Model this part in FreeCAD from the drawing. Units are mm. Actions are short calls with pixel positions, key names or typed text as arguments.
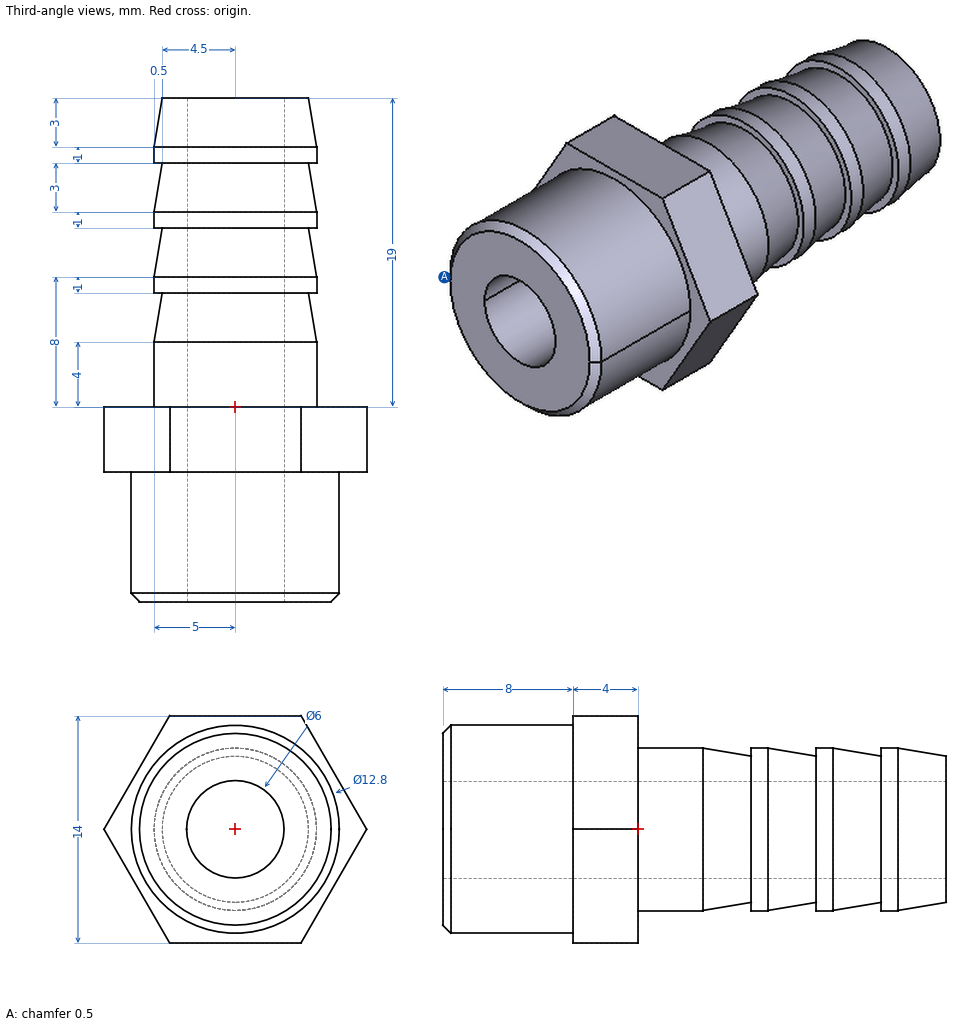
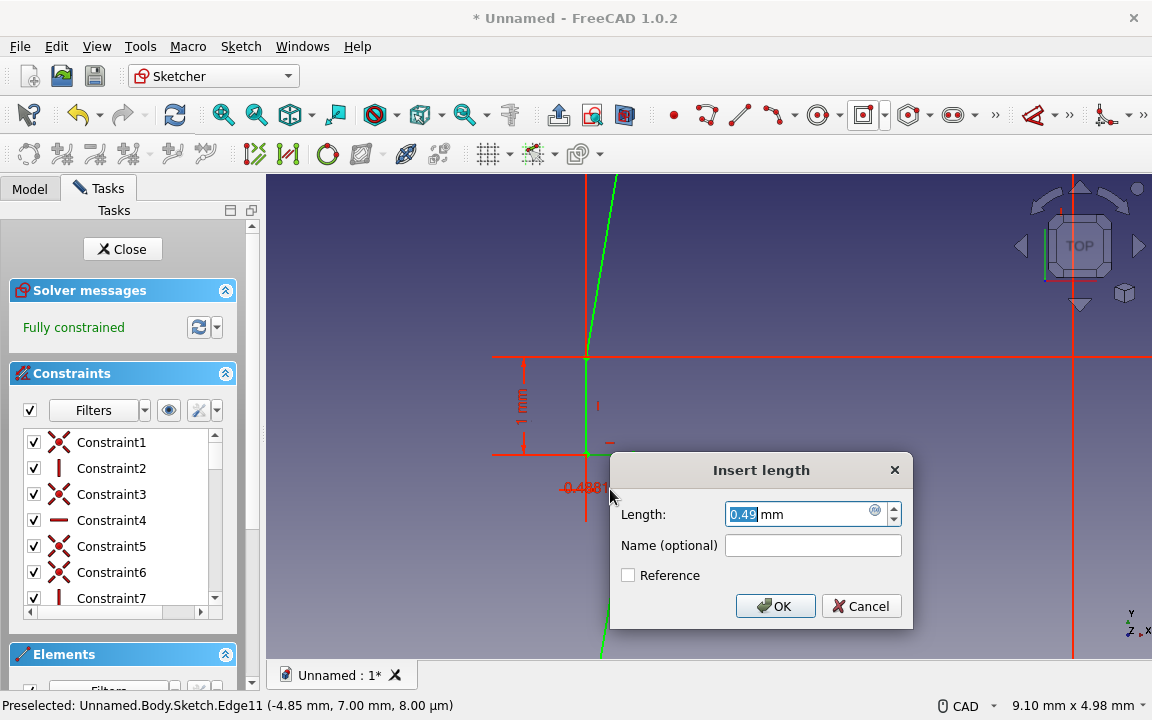
text(0.5)
key(Return)
key(Escape)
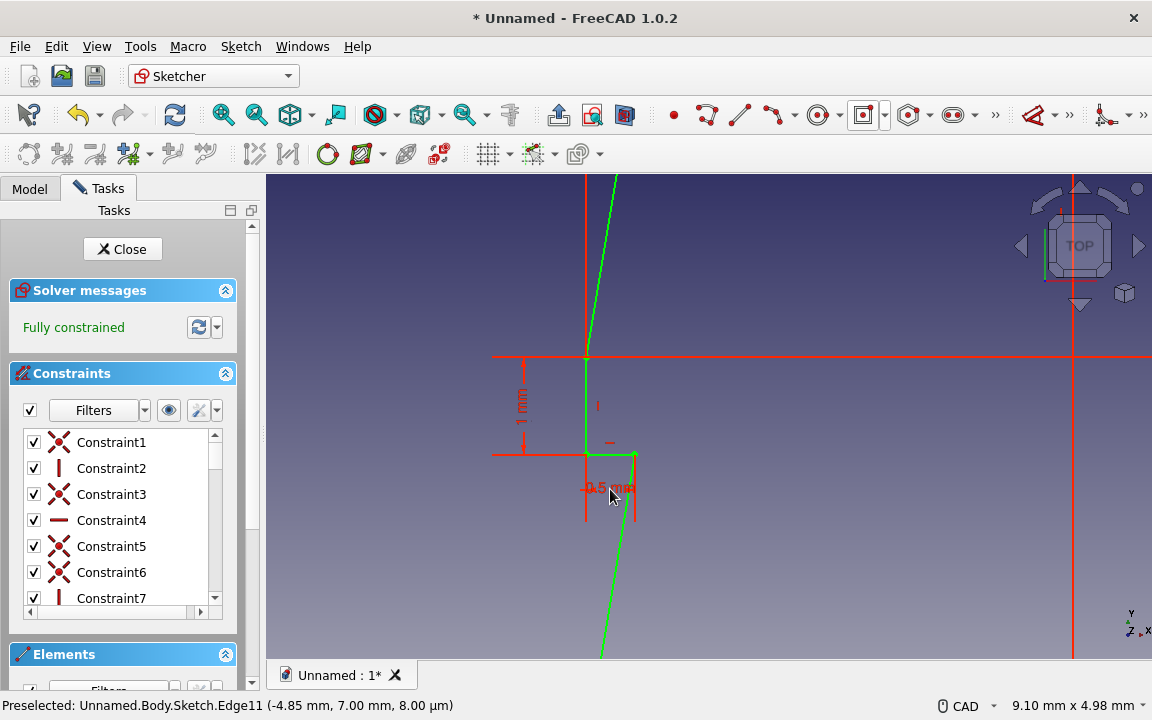
click(123, 249)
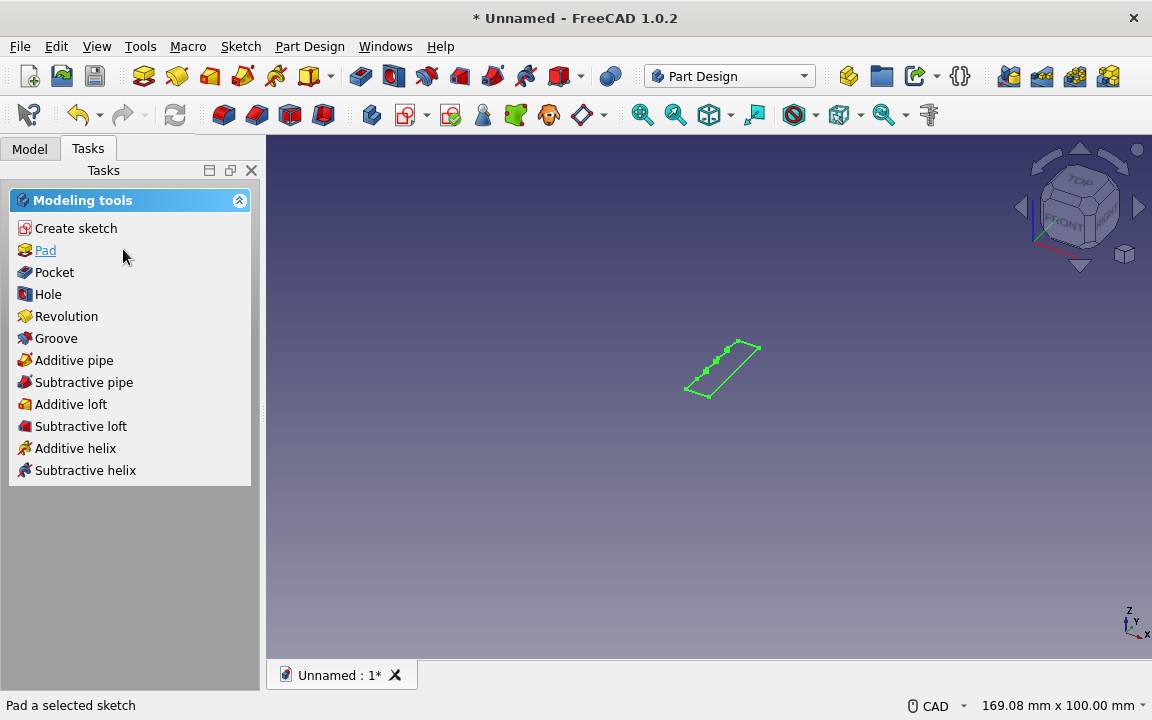
click(177, 76)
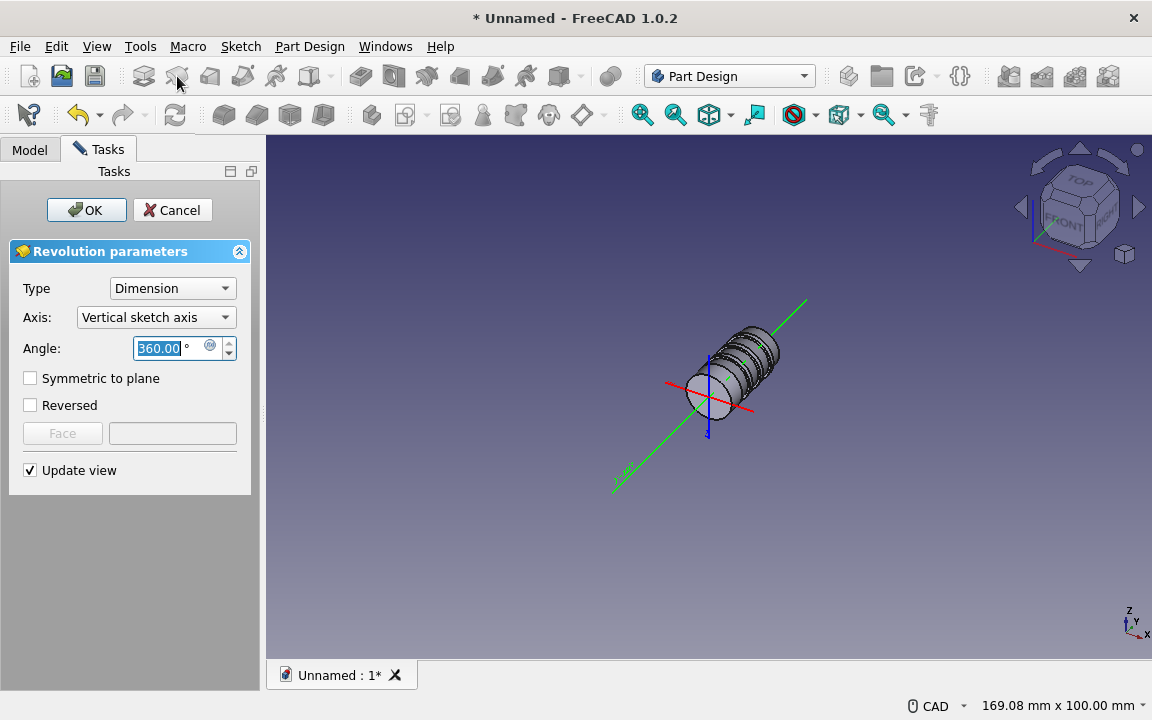
click(87, 210)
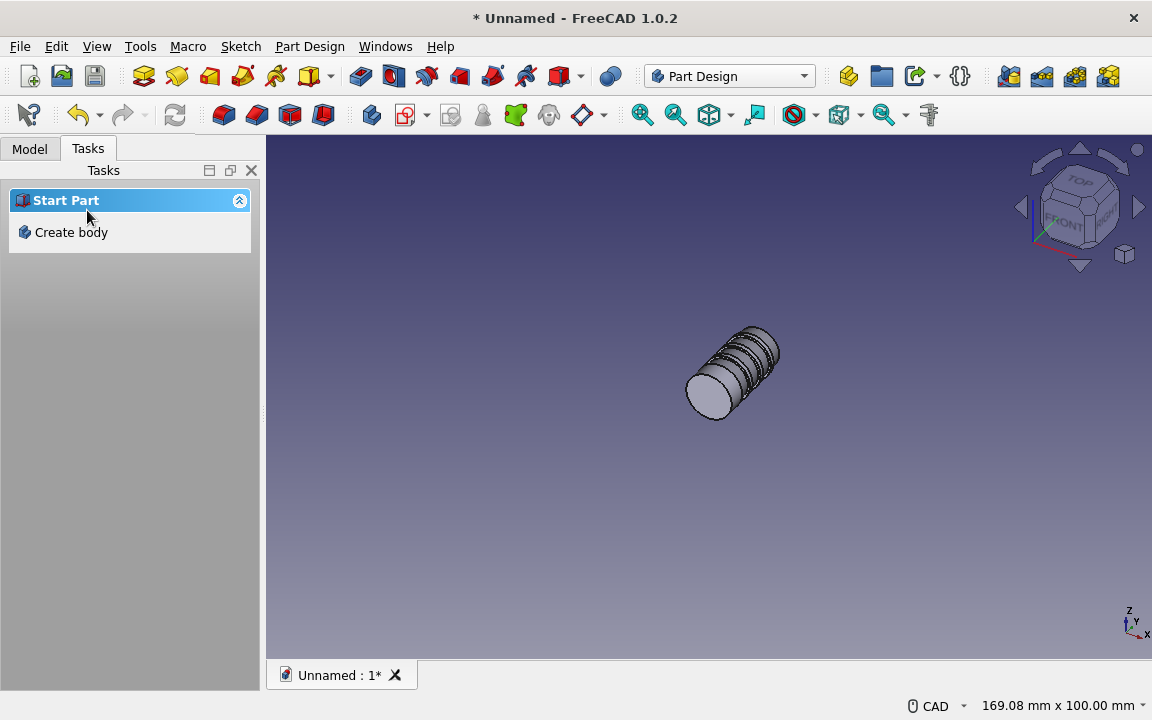
click(643, 116)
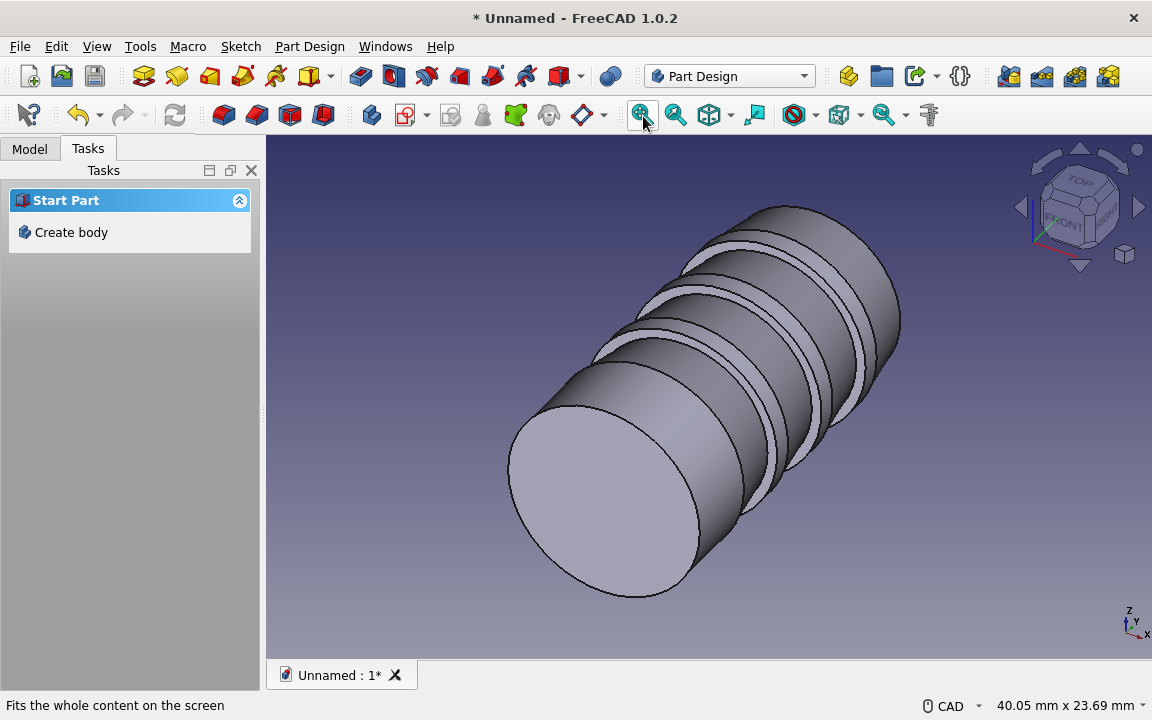
click(604, 500)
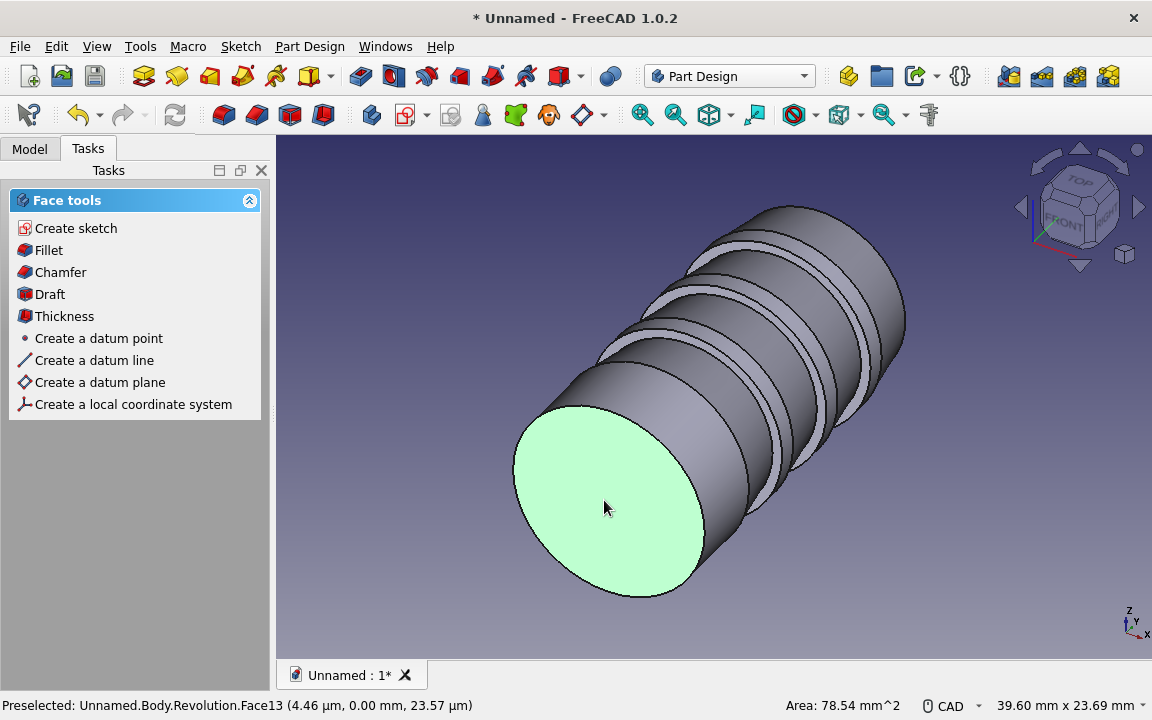
click(404, 116)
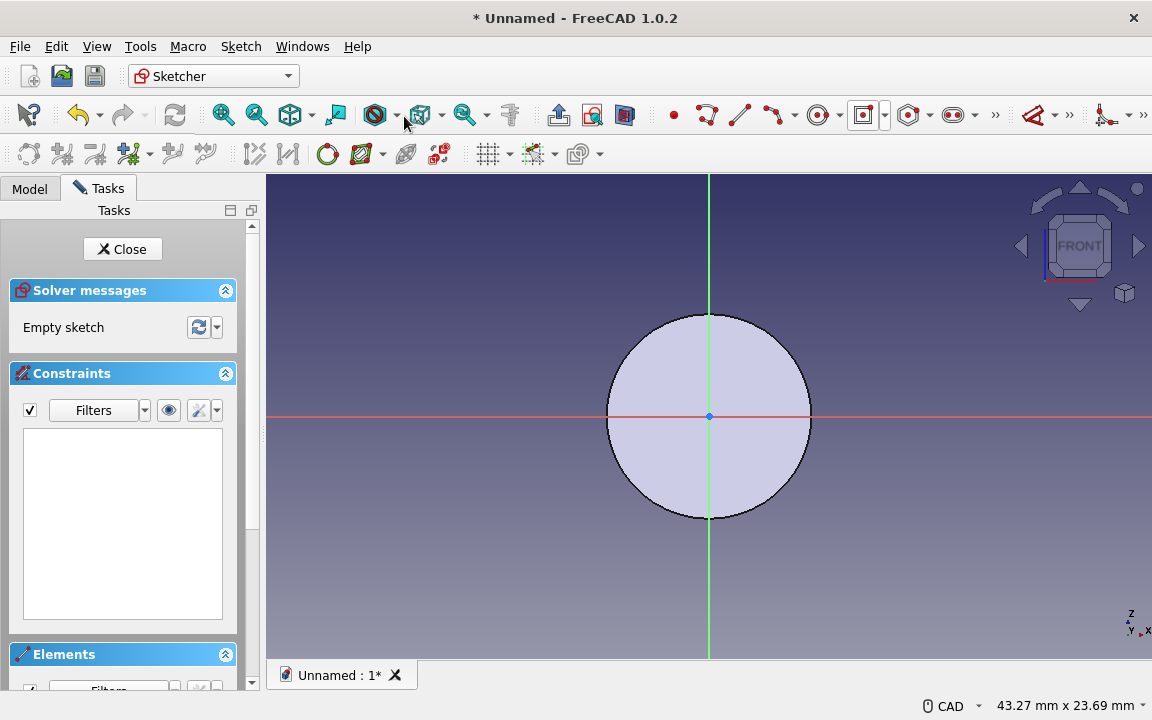
click(908, 116)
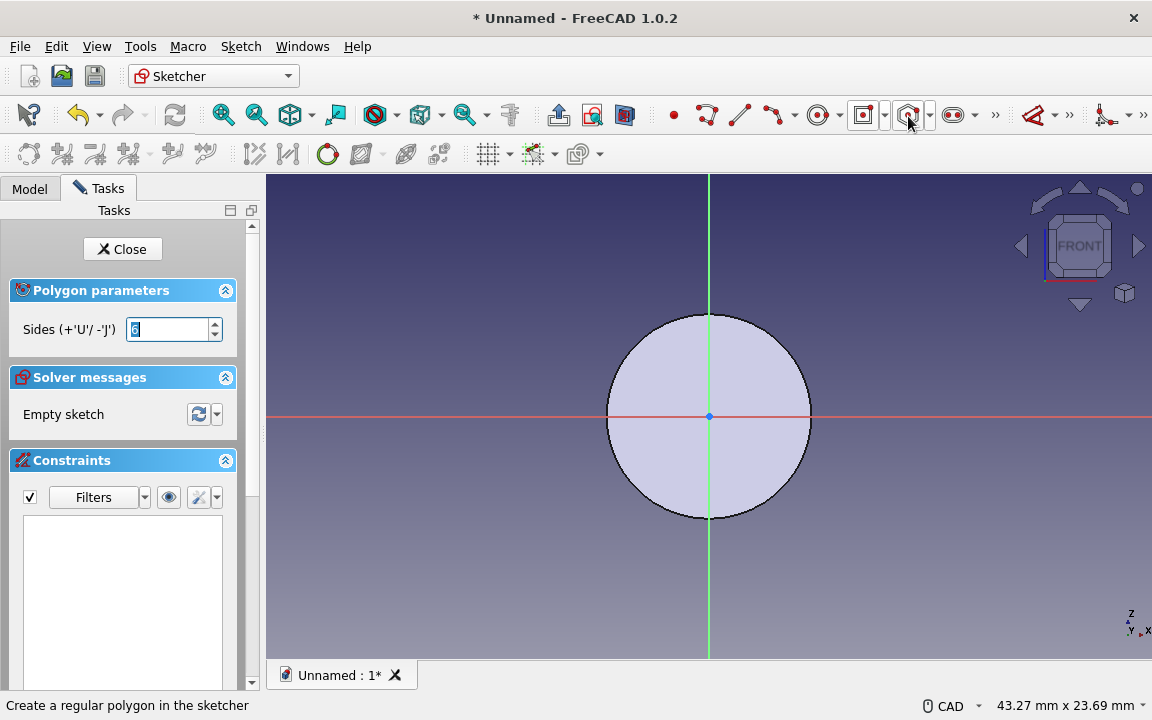
click(709, 417)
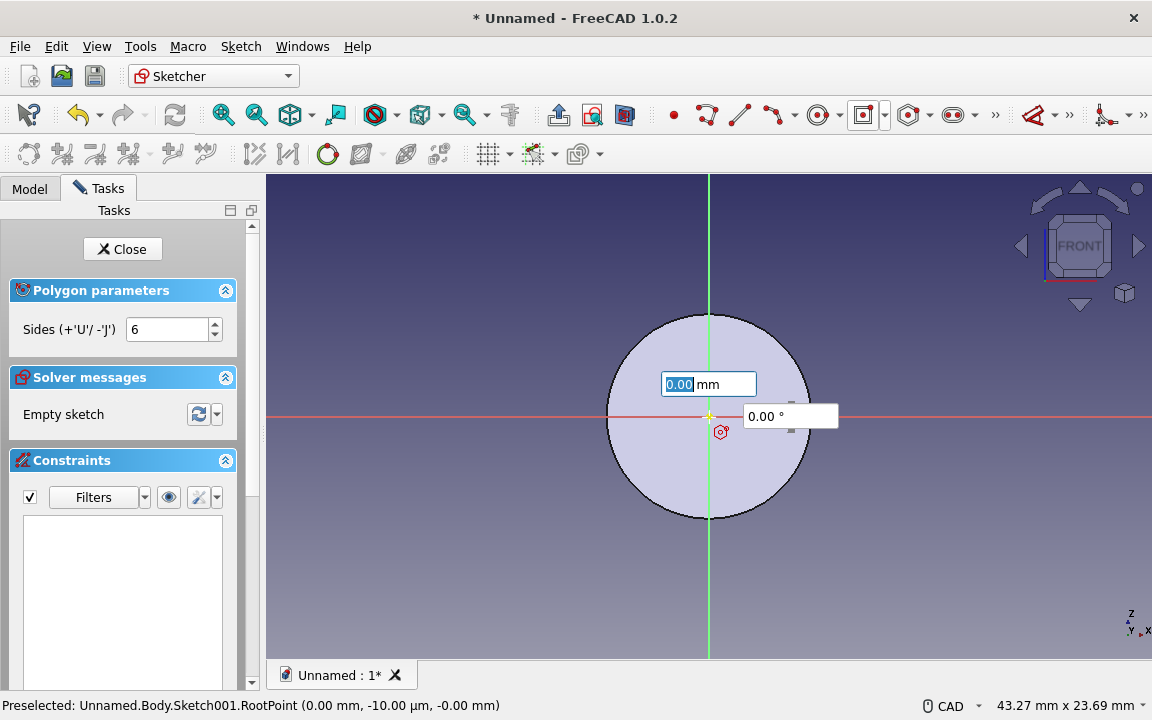
click(875, 417)
right_click(875, 417)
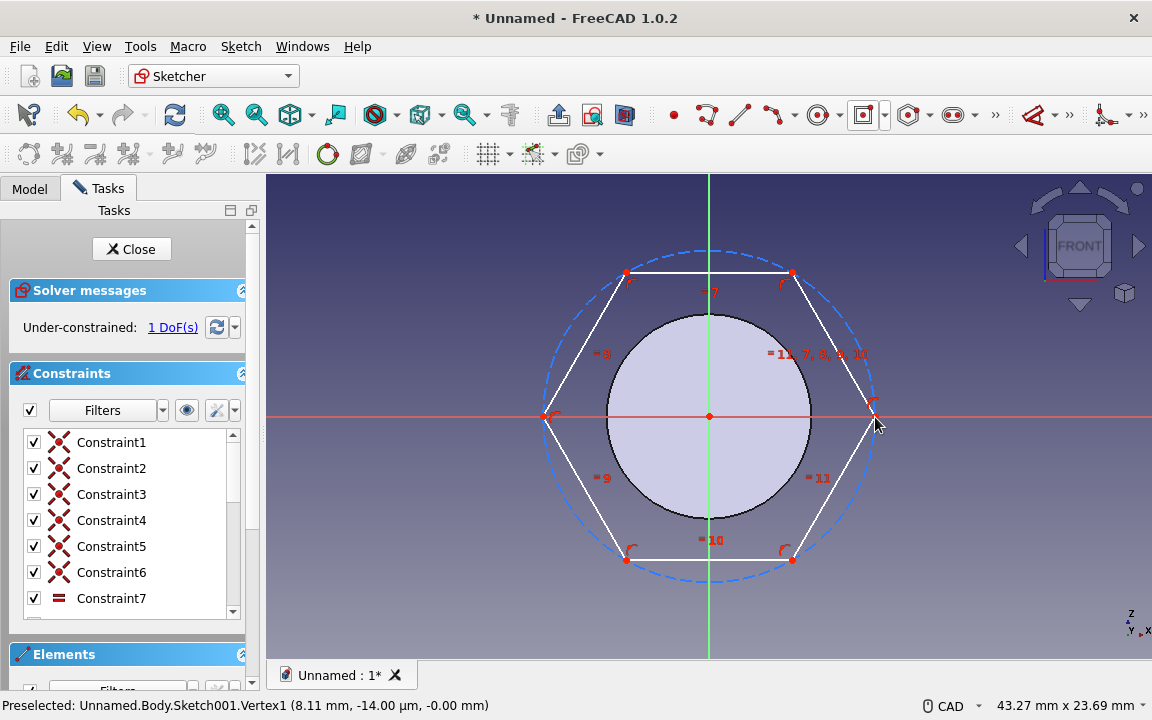
click(1032, 116)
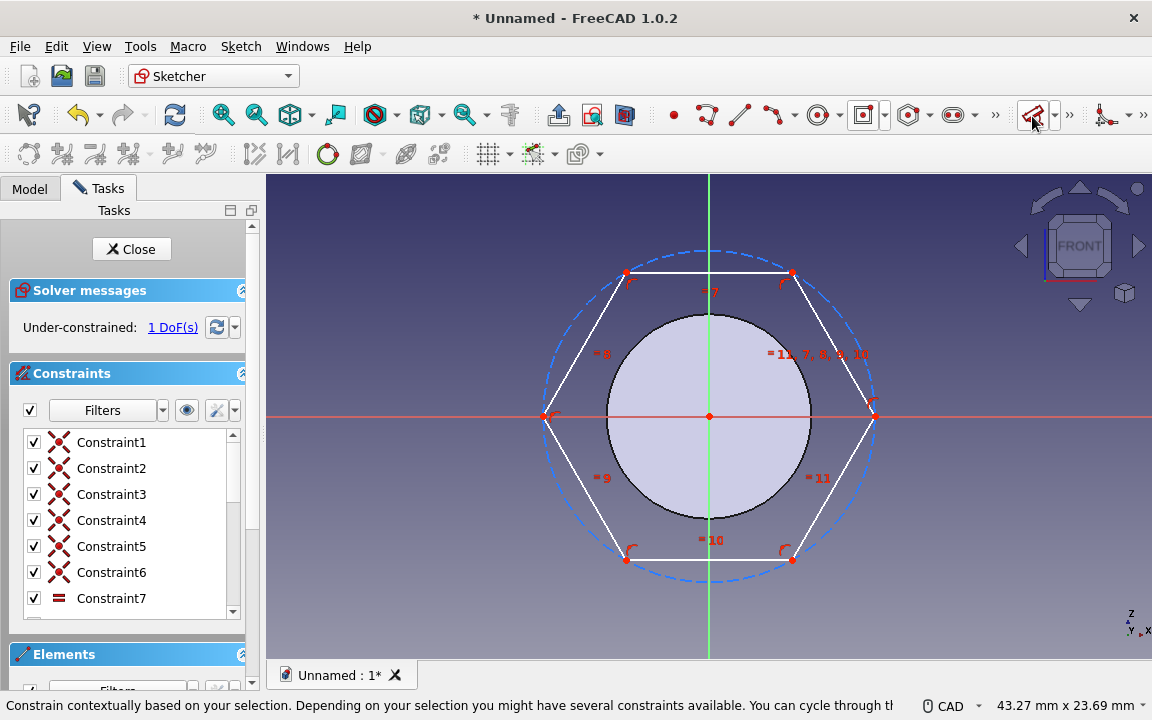
click(626, 560)